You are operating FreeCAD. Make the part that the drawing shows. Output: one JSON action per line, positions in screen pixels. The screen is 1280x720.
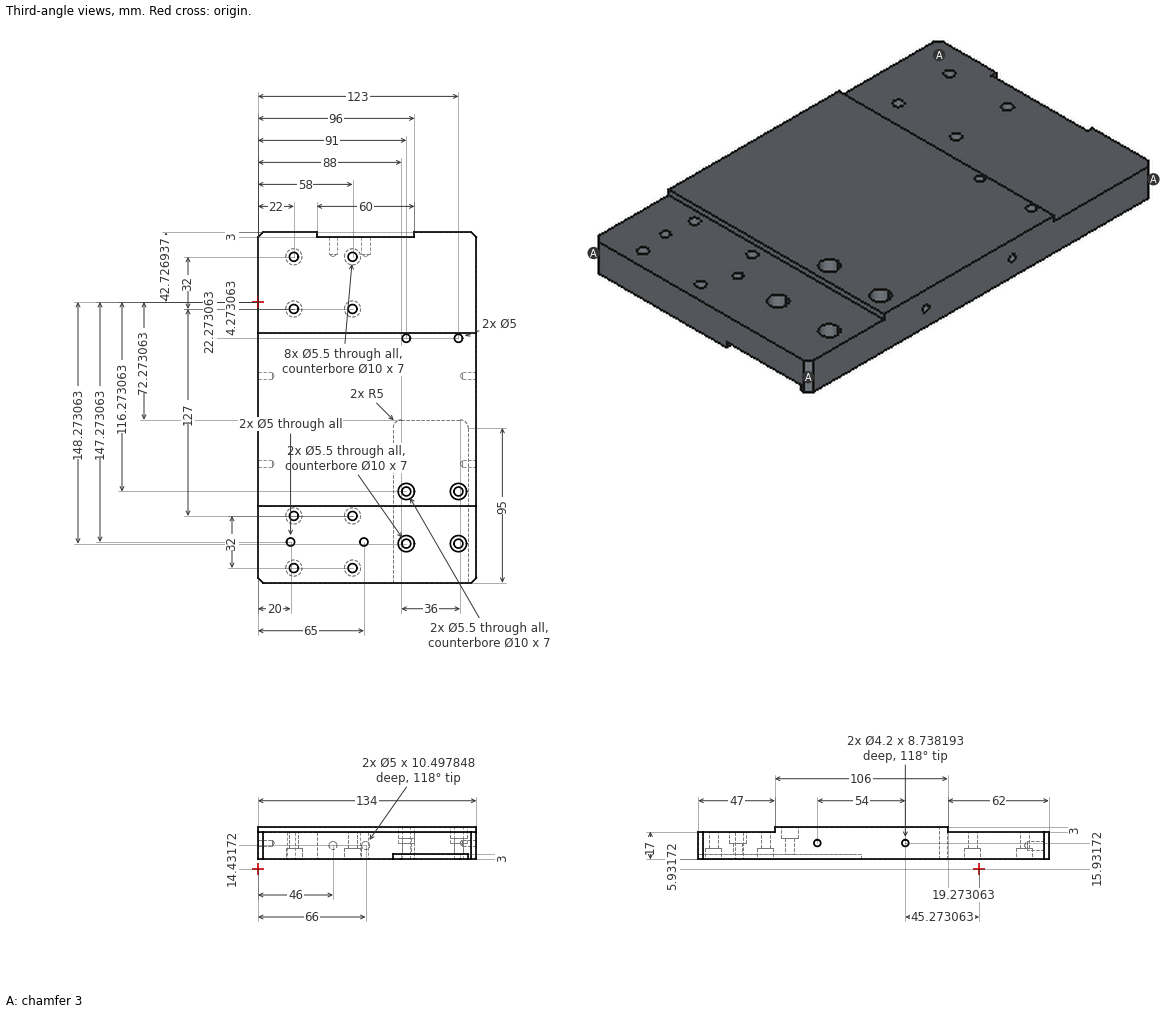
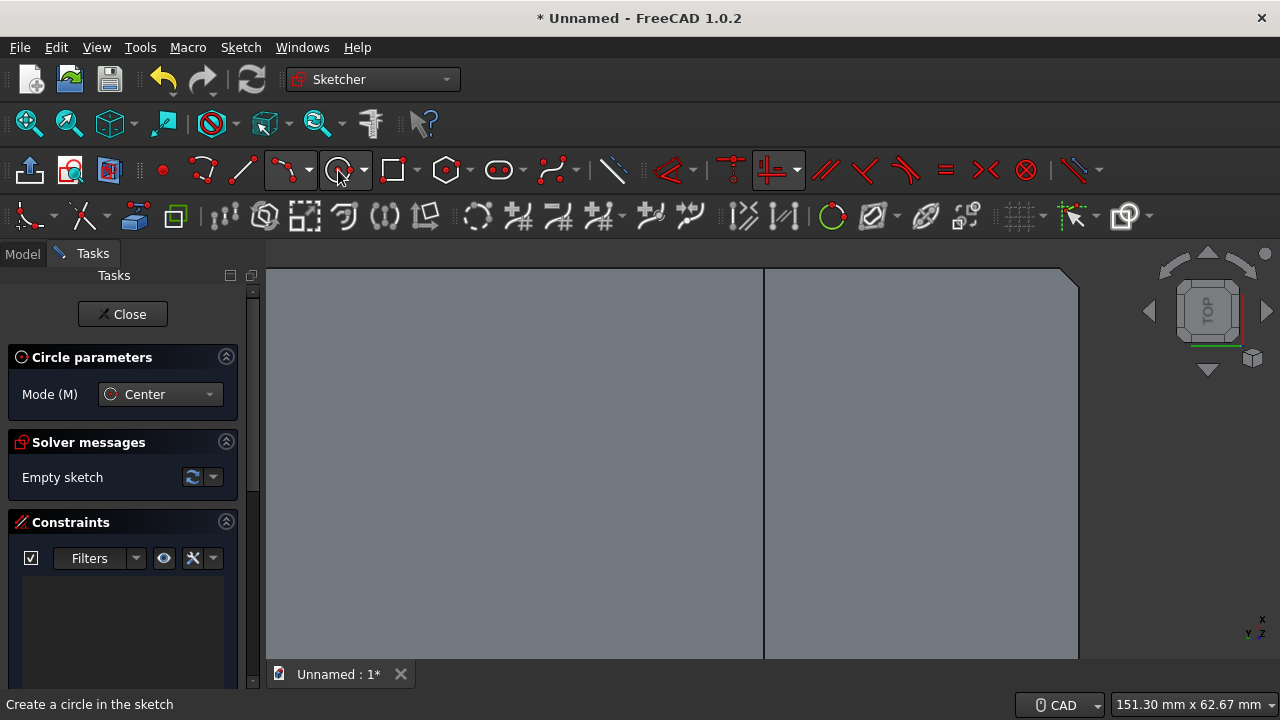
{"action": "scroll", "coordinate": [704, 556], "scroll_direction": "up", "scroll_amount": 2}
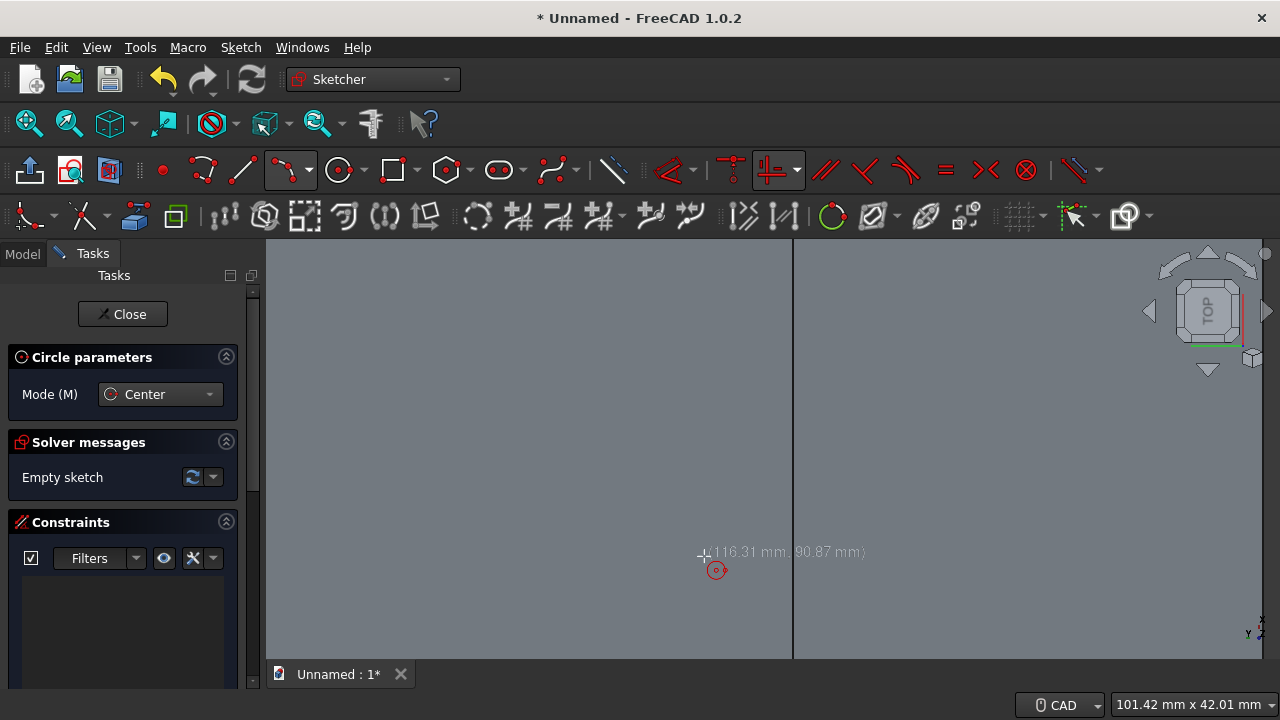
{"action": "left_click", "coordinate": [703, 556]}
{"action": "mouse_move", "coordinate": [723, 536]}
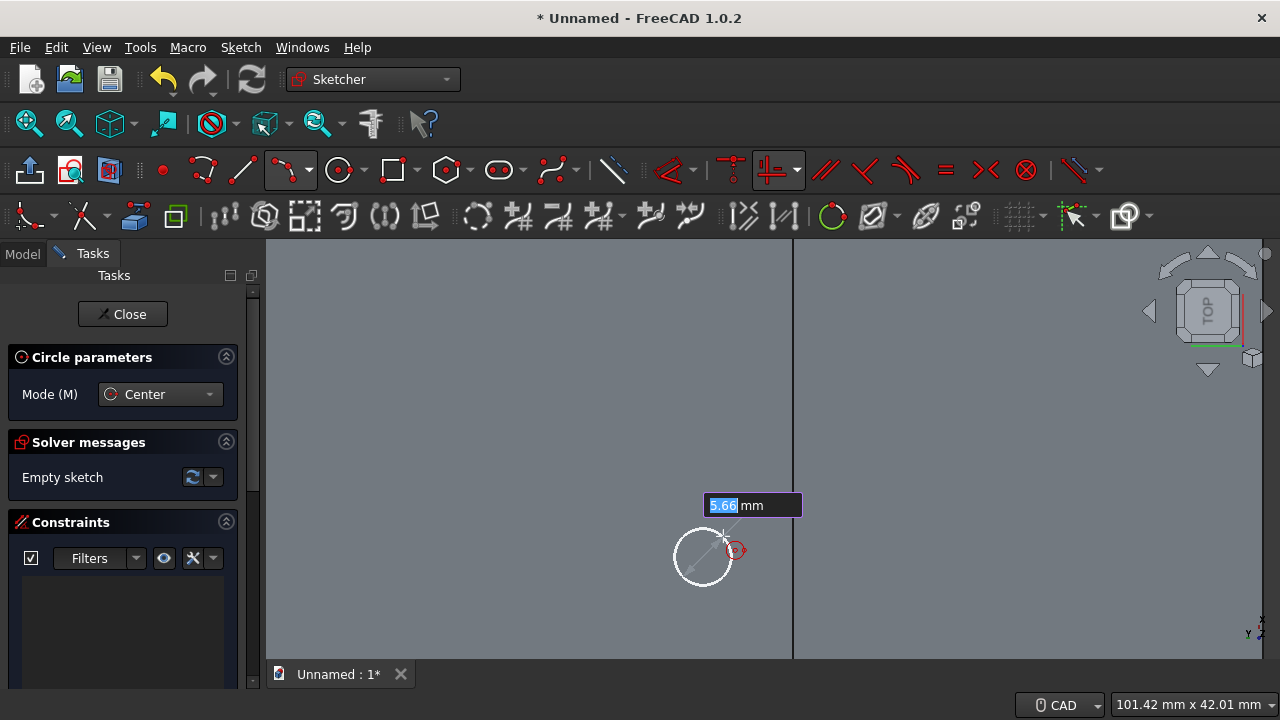
{"action": "type", "text": "5.5"}
{"action": "key", "text": "Return"}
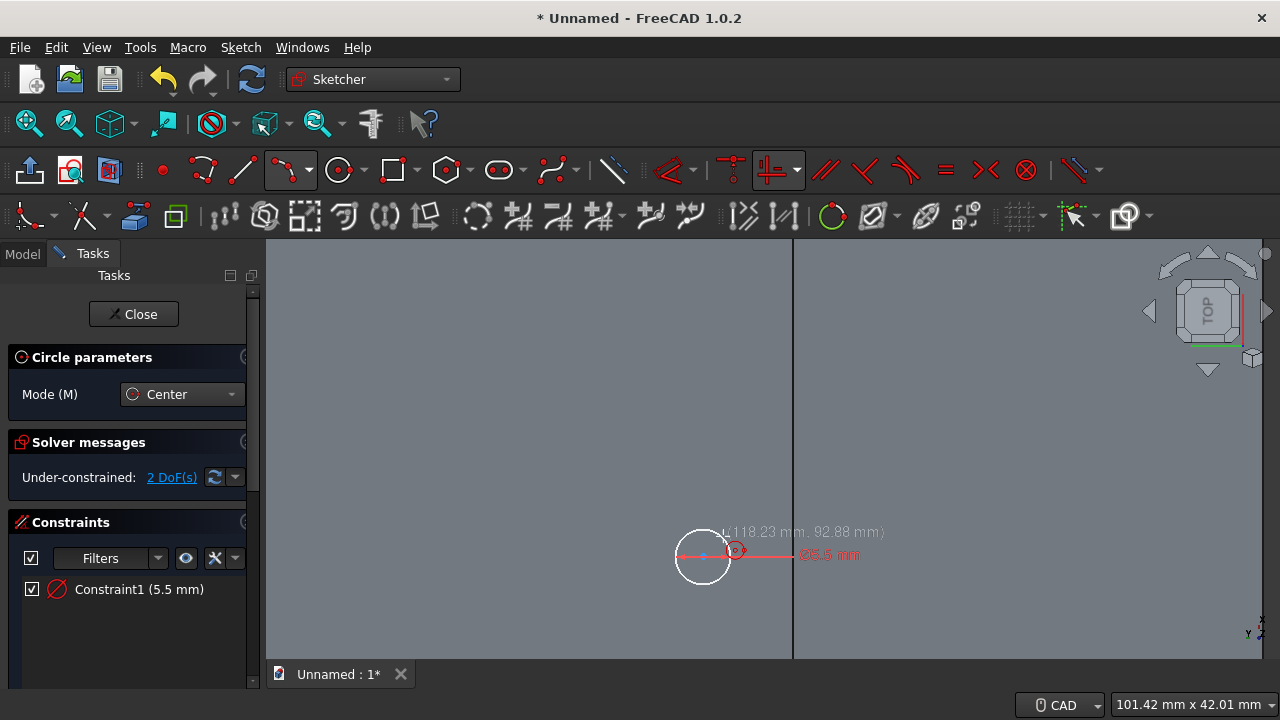
{"action": "scroll", "coordinate": [707, 557], "scroll_direction": "down", "scroll_amount": 2}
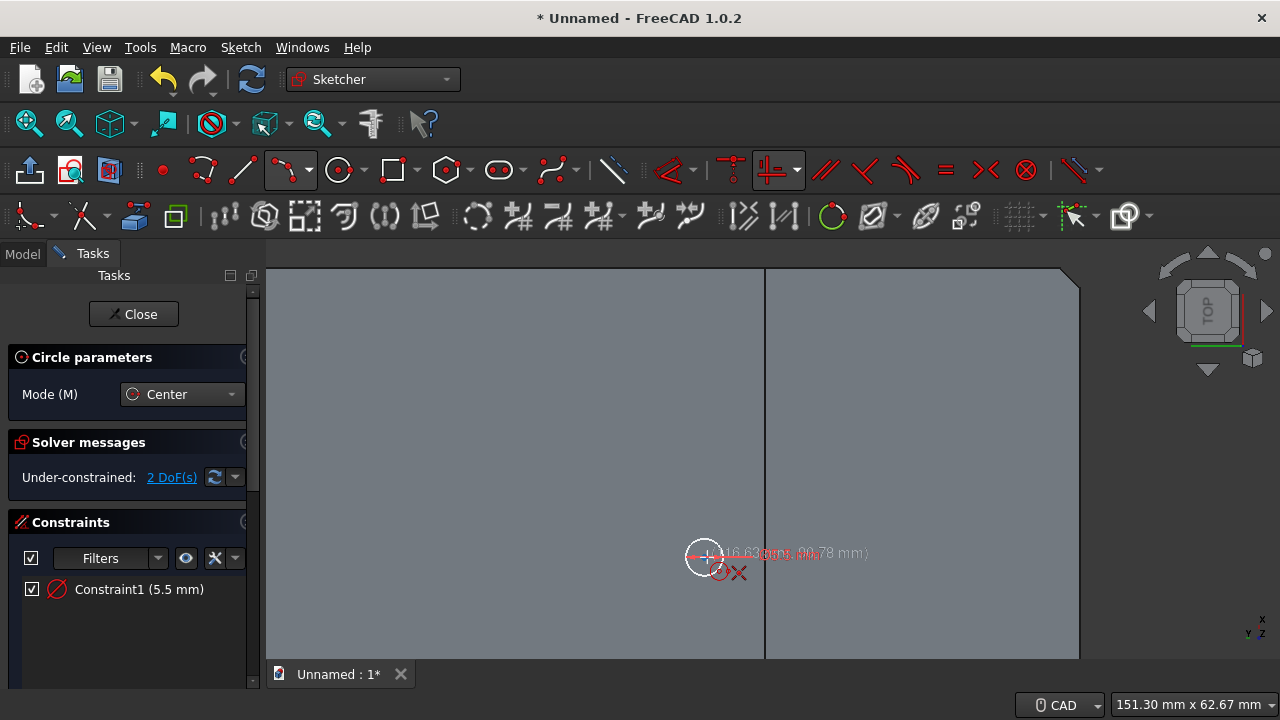
{"action": "scroll", "coordinate": [705, 342], "scroll_direction": "up", "scroll_amount": 2}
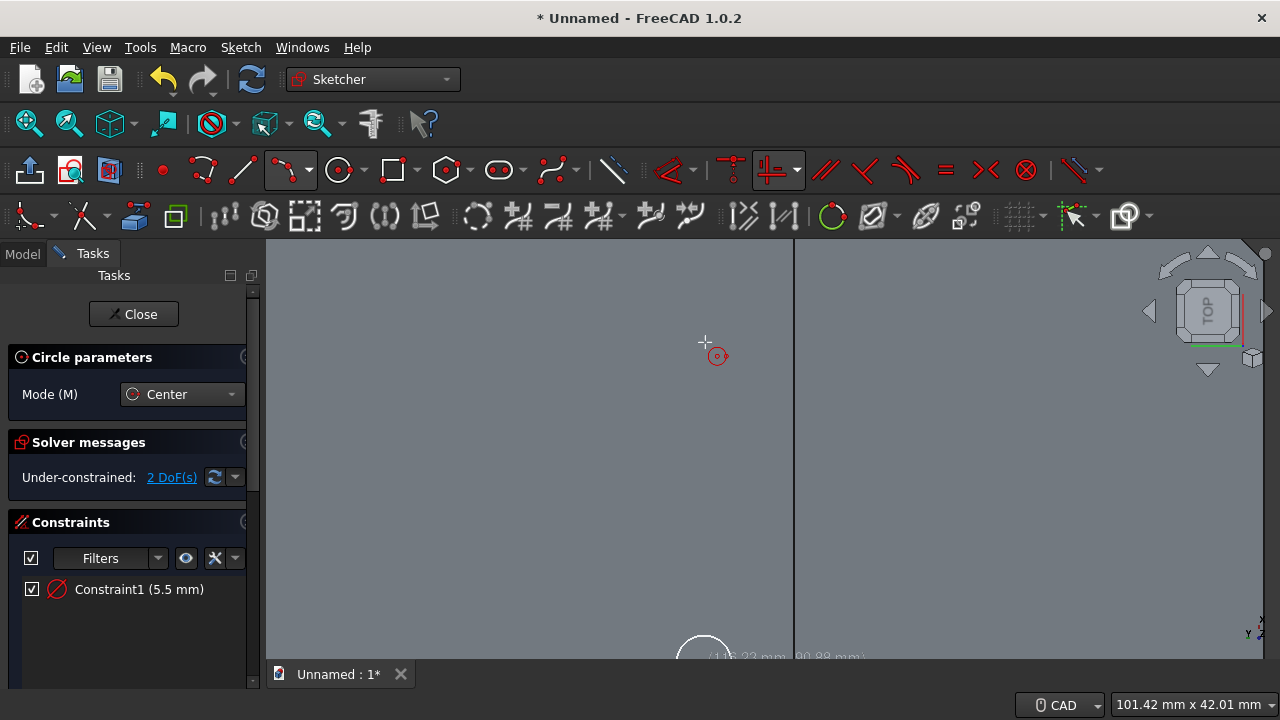
{"action": "left_click", "coordinate": [704, 342]}
{"action": "mouse_move", "coordinate": [724, 322]}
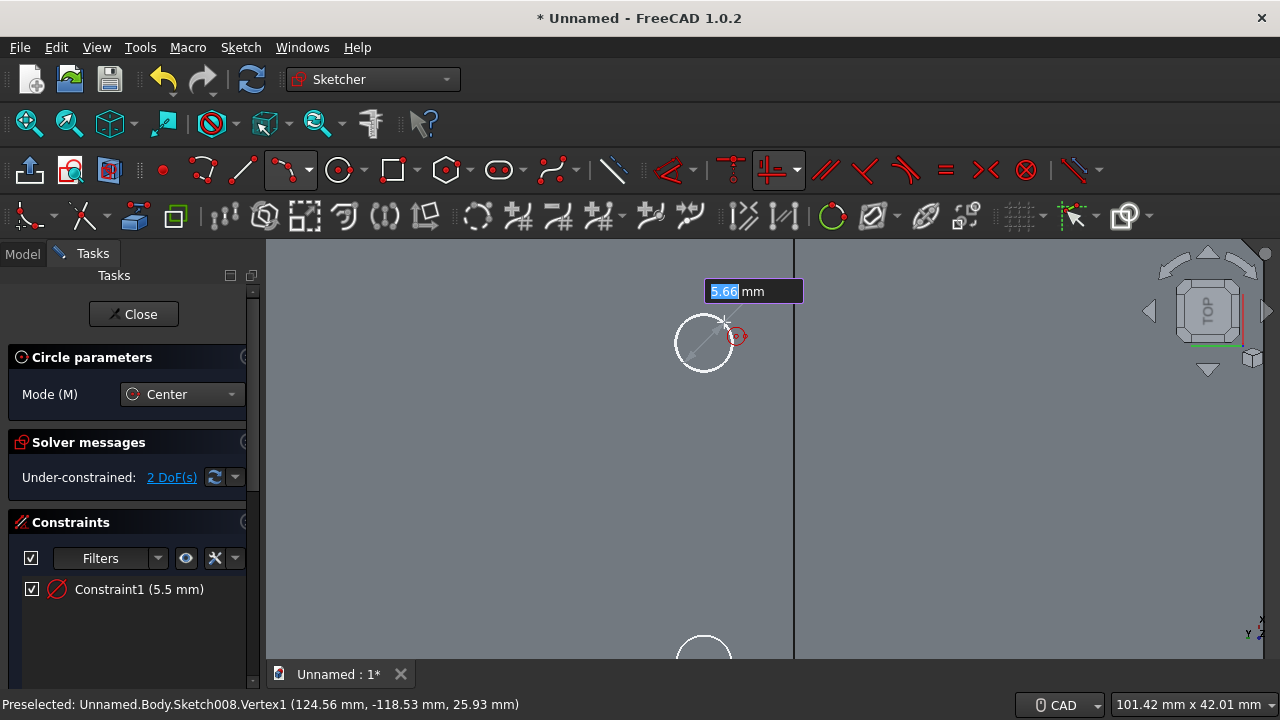
{"action": "type", "text": "5.5"}
{"action": "key", "text": "Return"}
{"action": "key", "text": "Escape"}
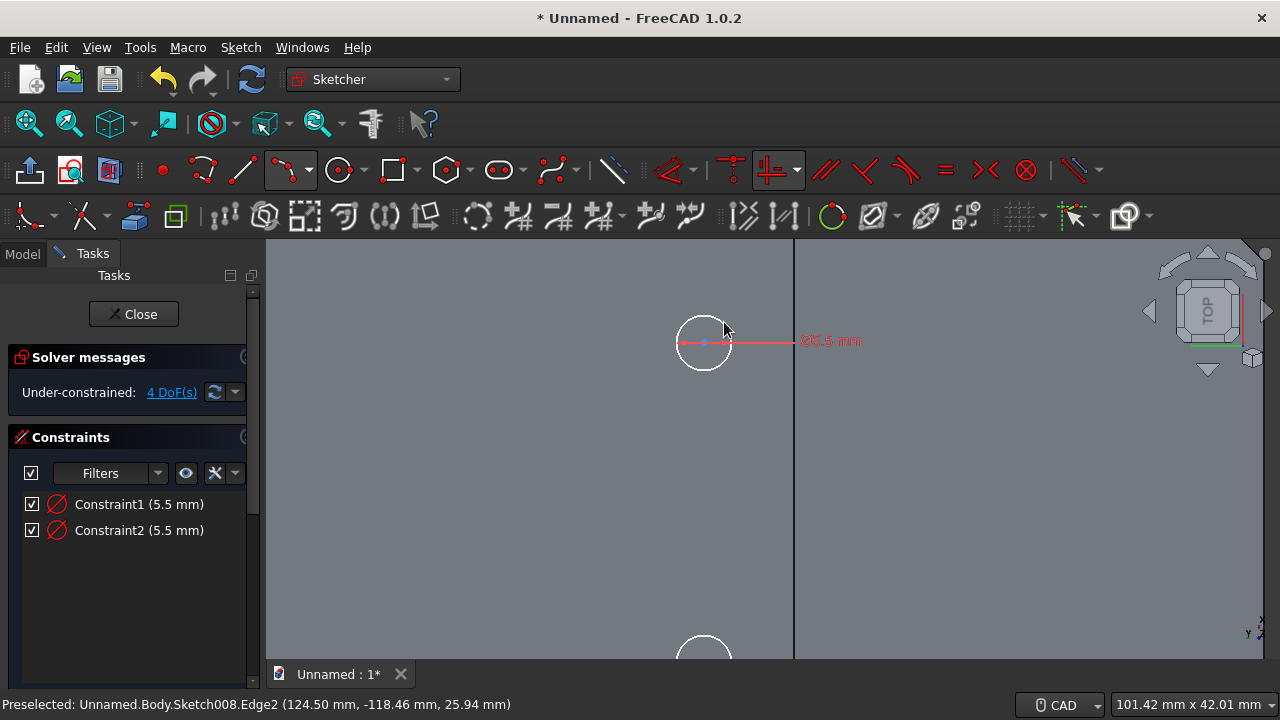
{"action": "scroll", "coordinate": [705, 342], "scroll_direction": "down", "scroll_amount": 2}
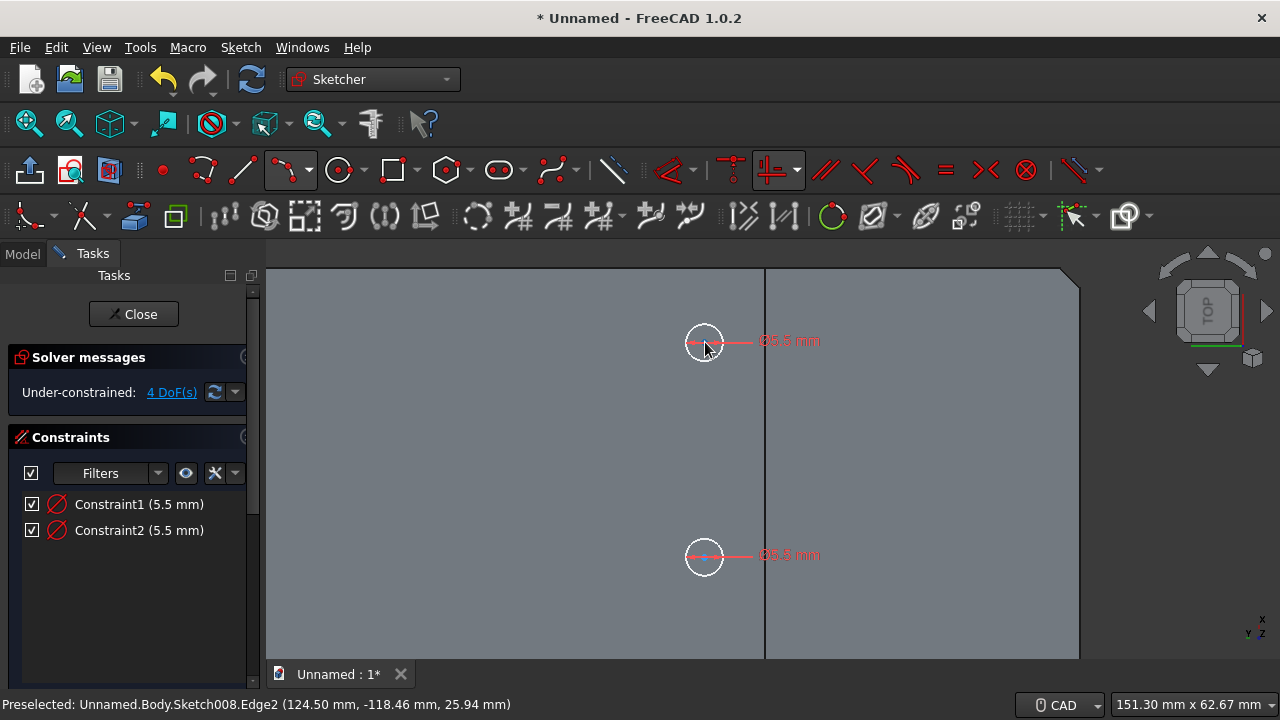
{"action": "left_click", "coordinate": [704, 557]}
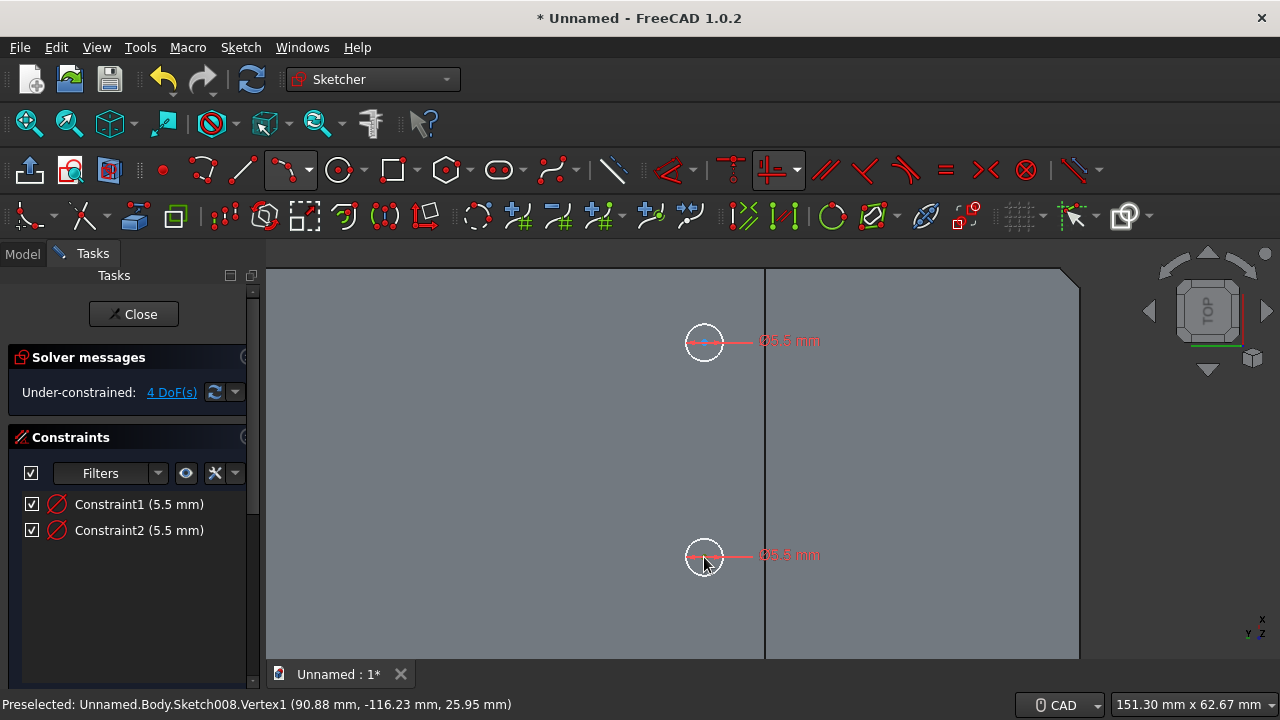
{"action": "left_click", "coordinate": [704, 343]}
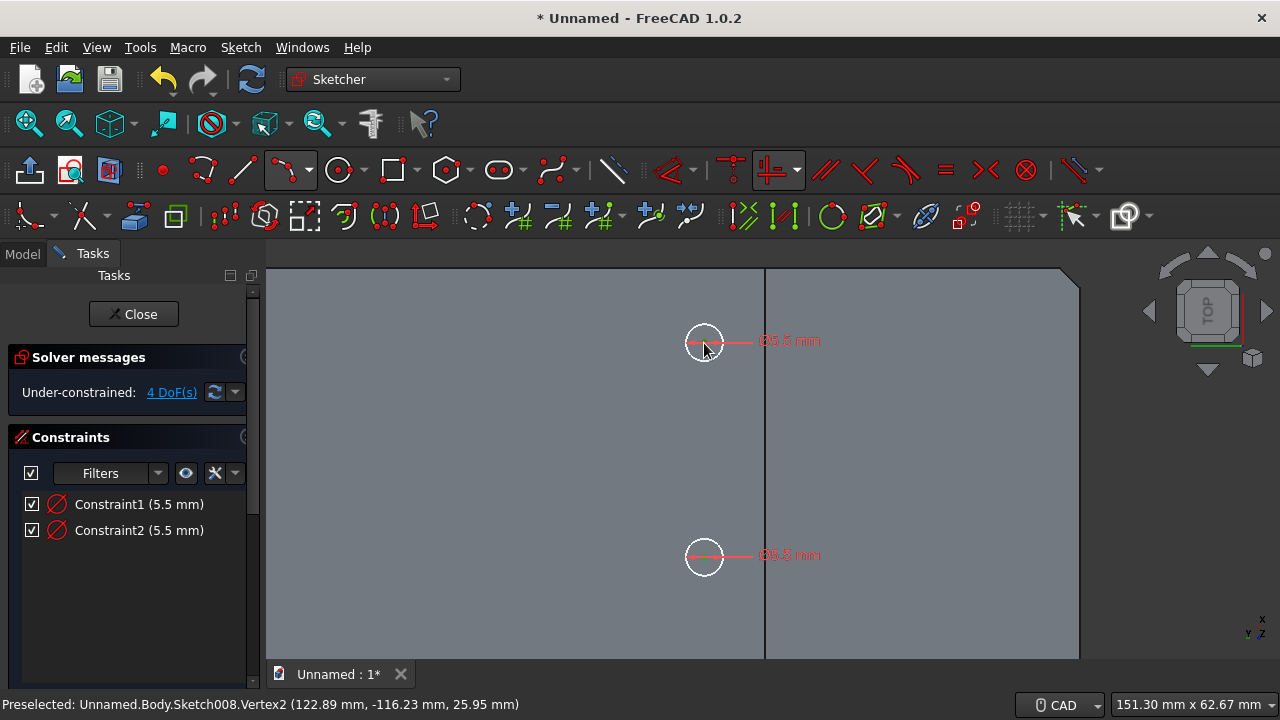
{"action": "key", "text": "v"}